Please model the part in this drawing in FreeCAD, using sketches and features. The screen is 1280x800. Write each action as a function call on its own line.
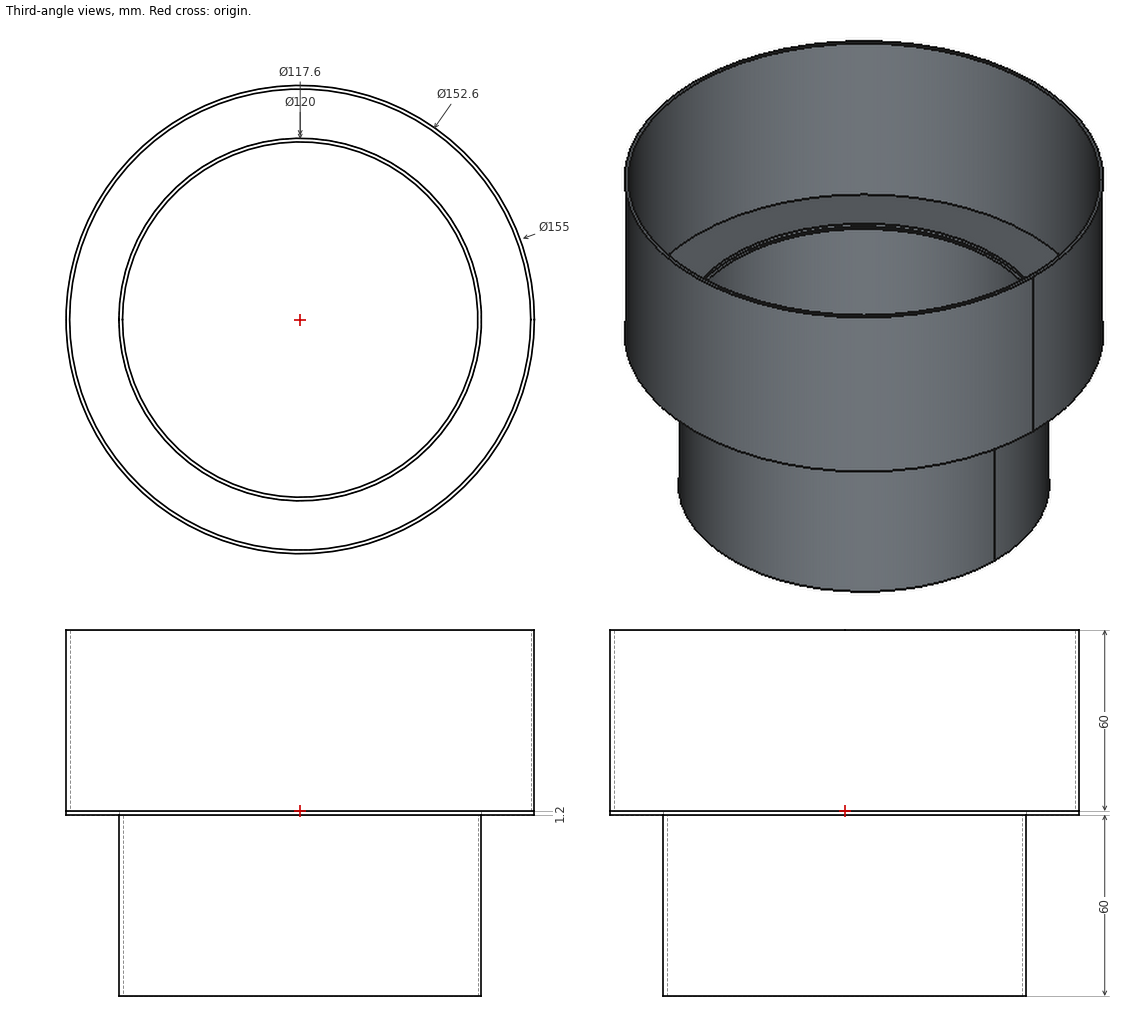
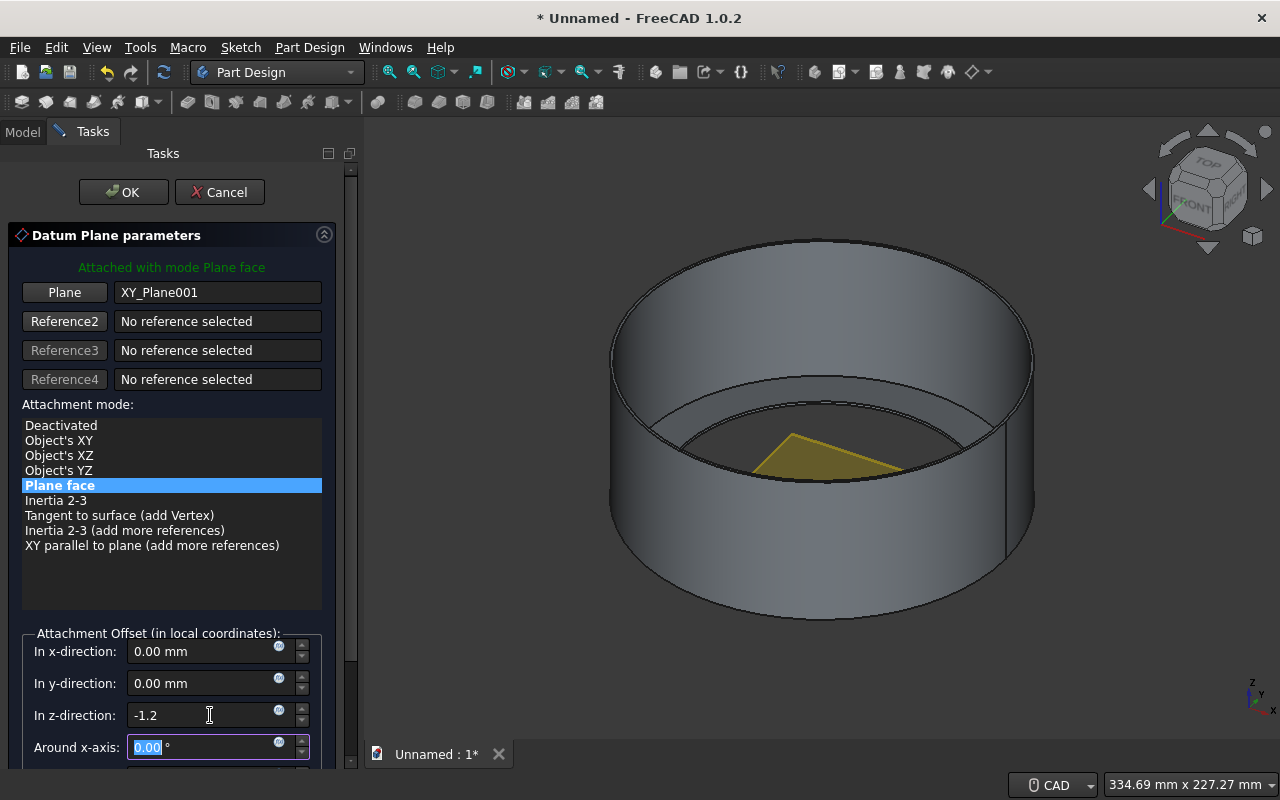
click(124, 192)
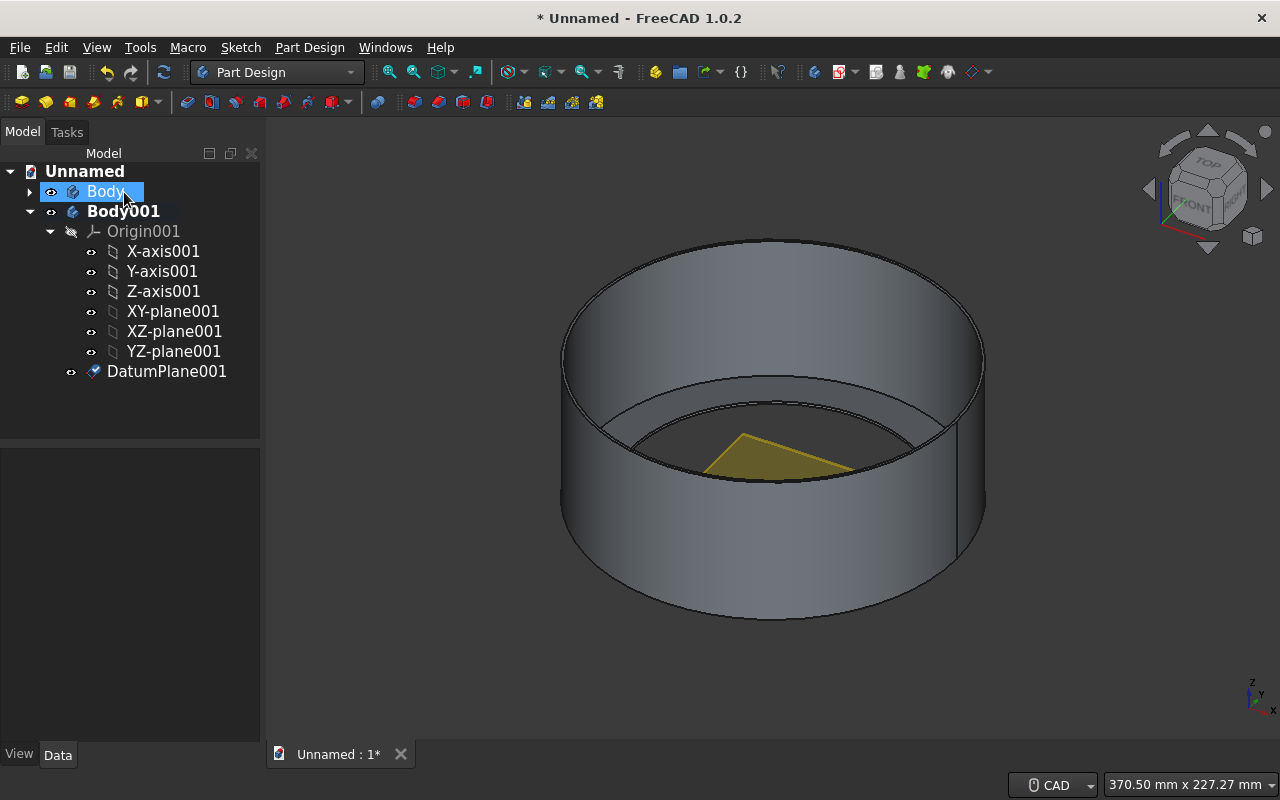
click(116, 372)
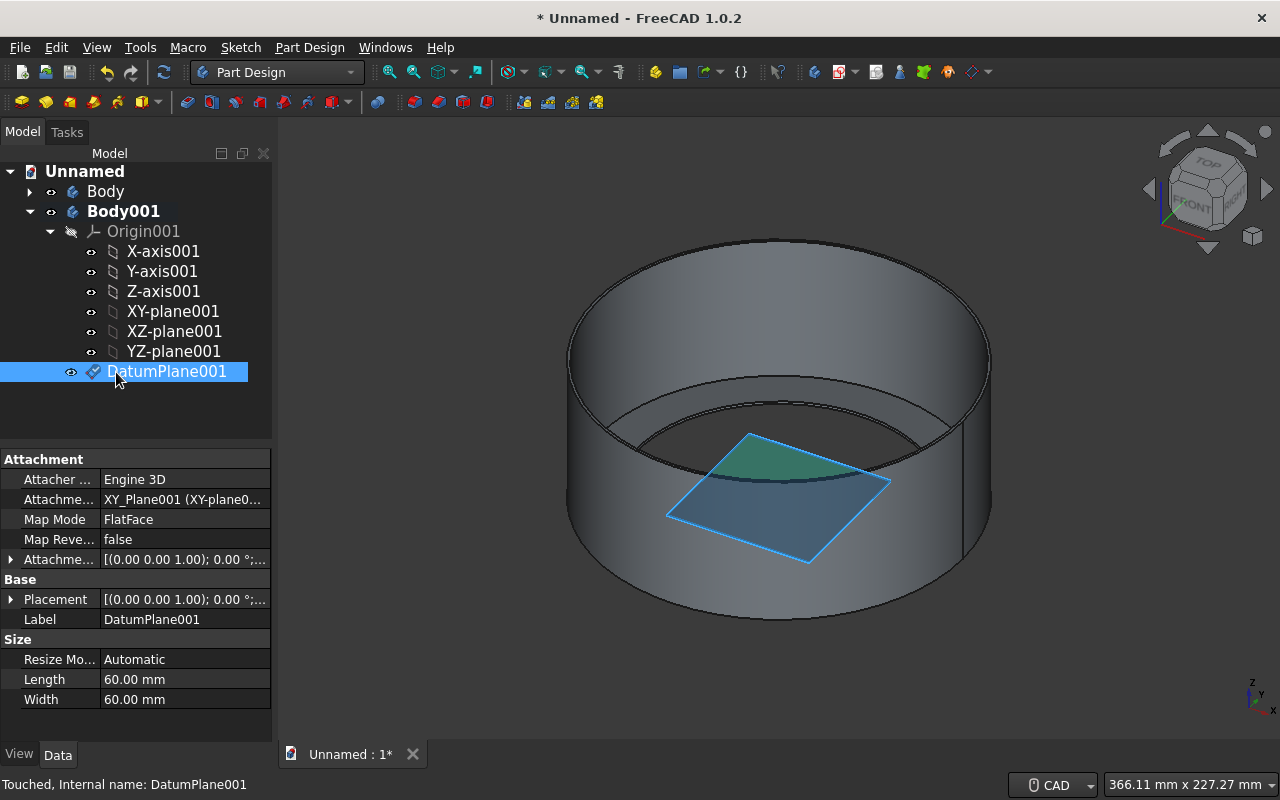
click(840, 72)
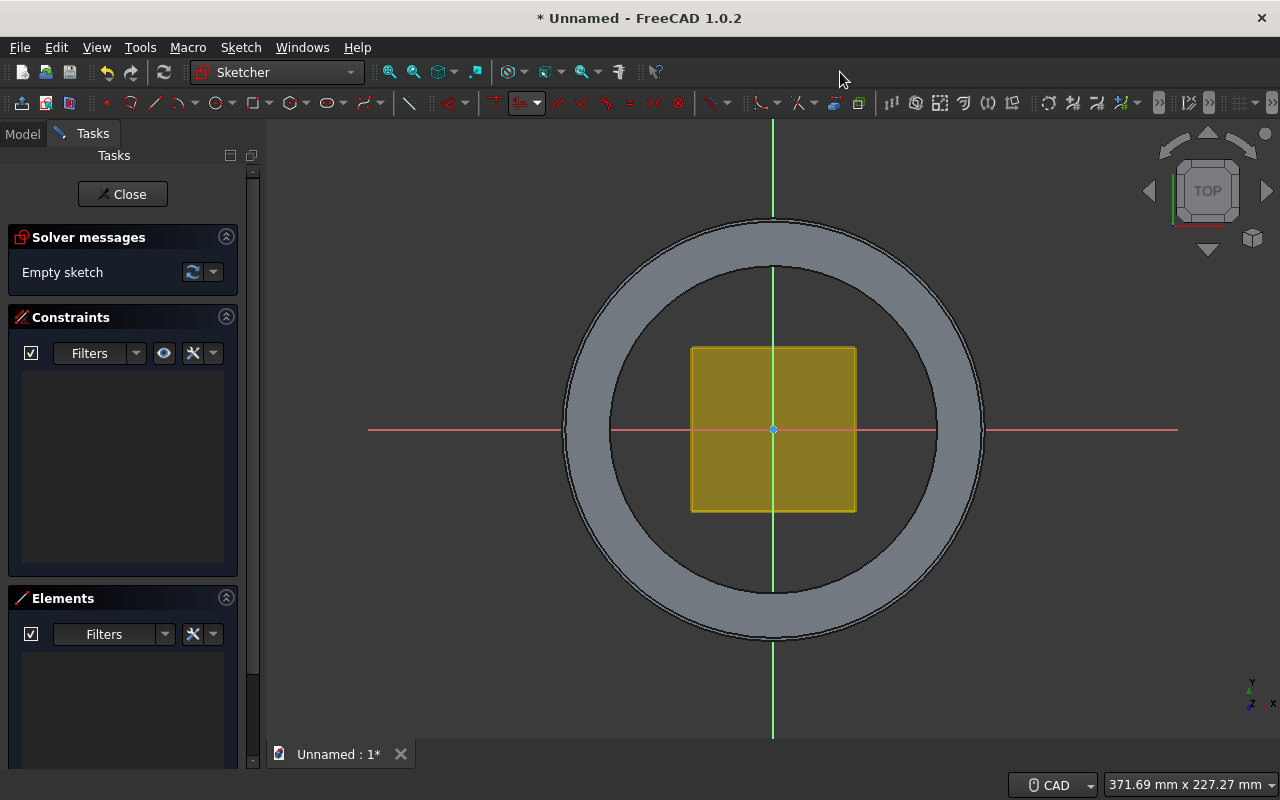
click(216, 104)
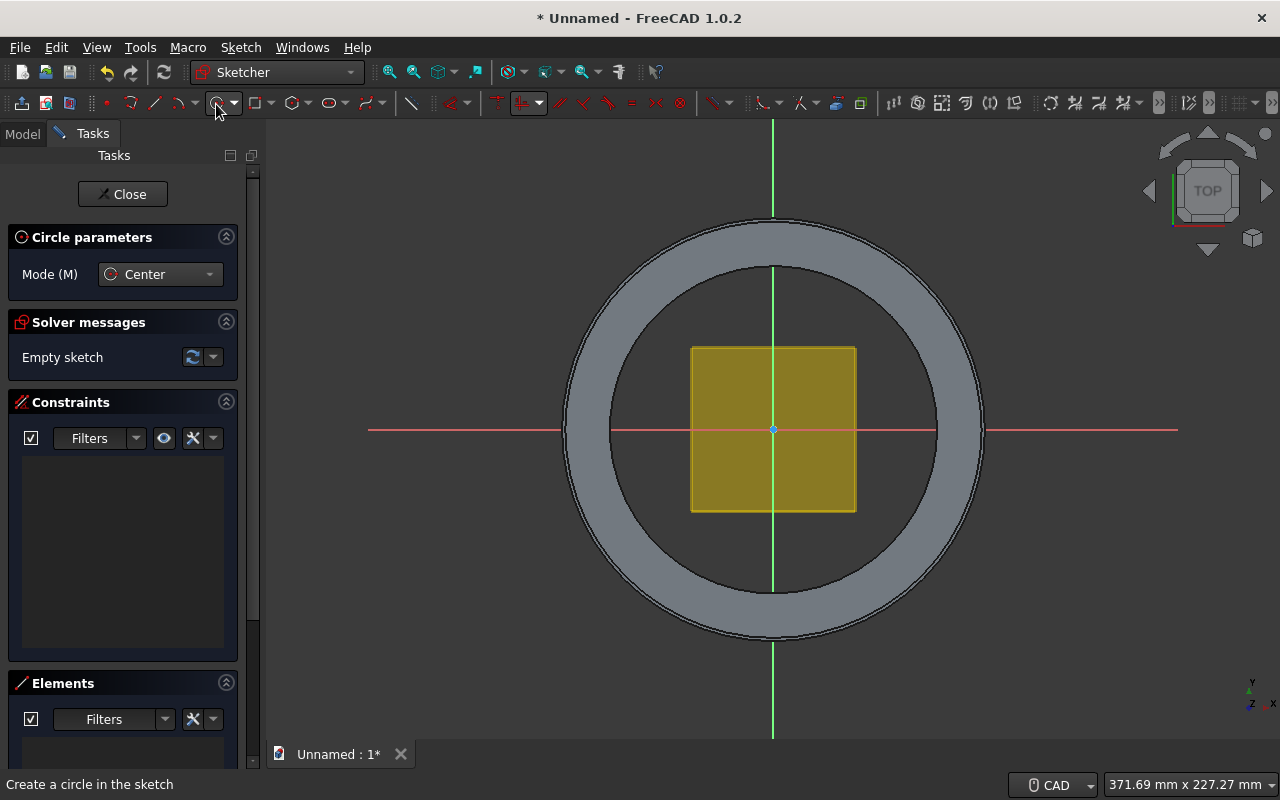
click(773, 430)
click(889, 314)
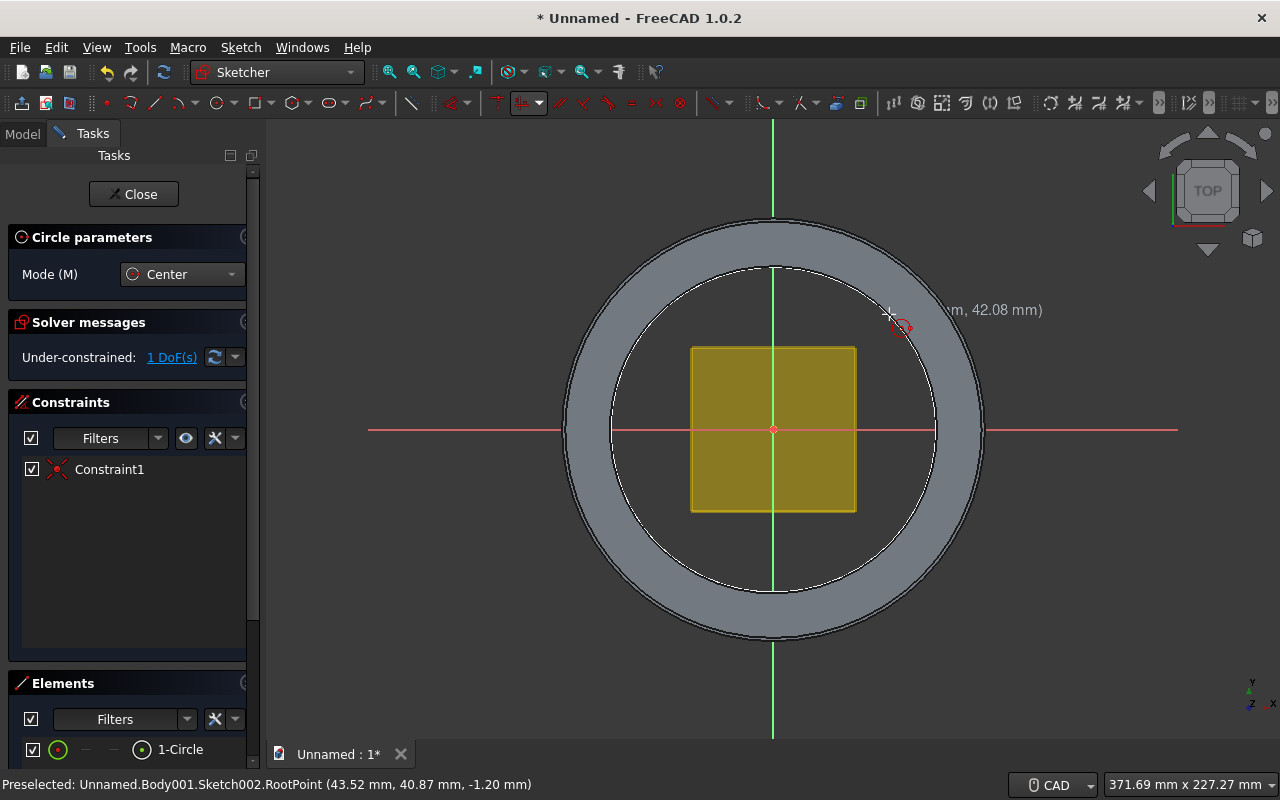
click(773, 430)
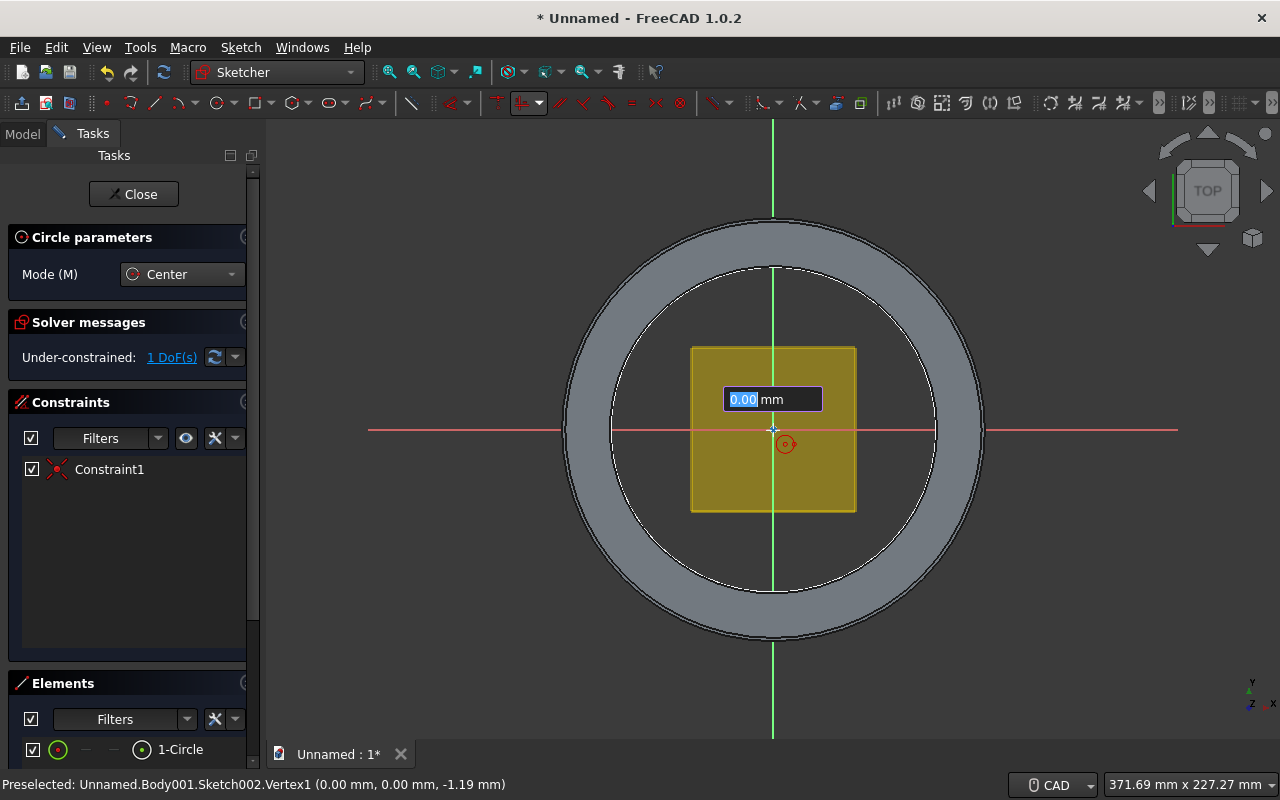
scroll(887, 316, up, 8)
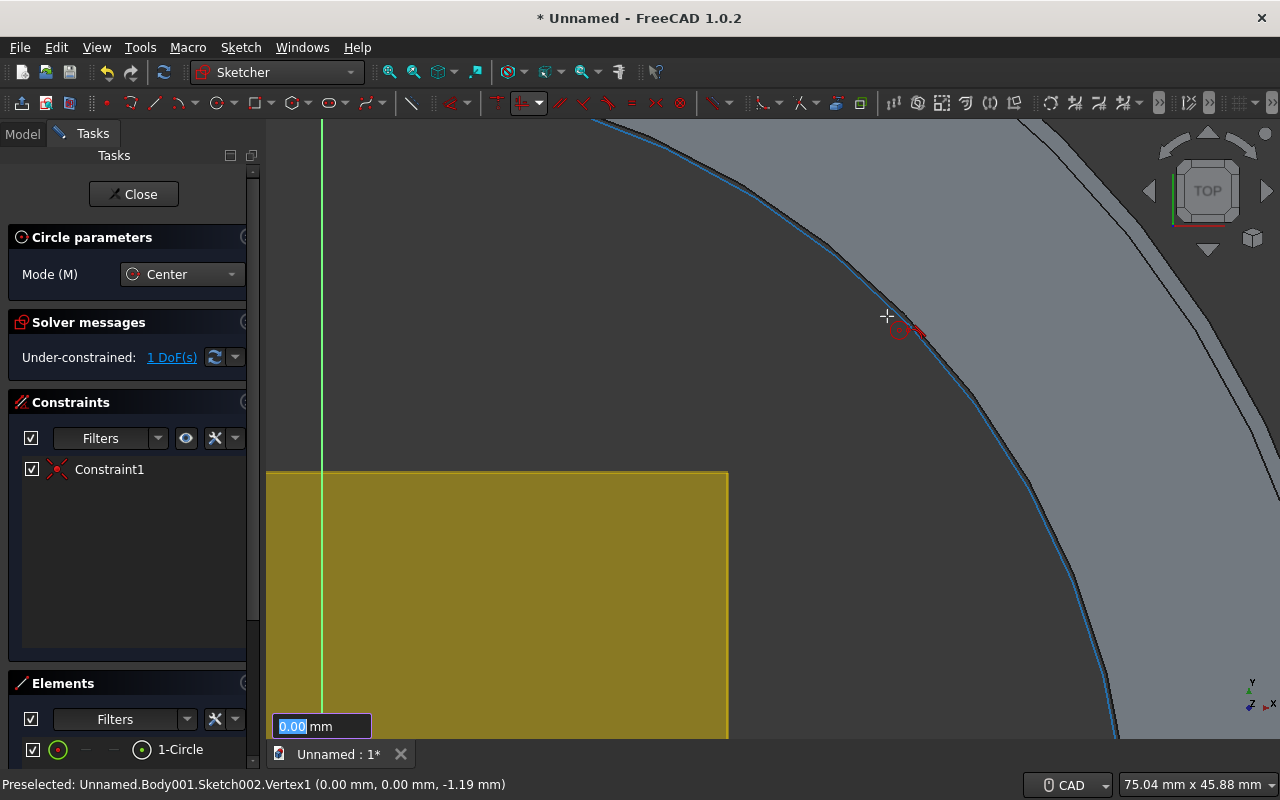
click(884, 317)
key(Escape)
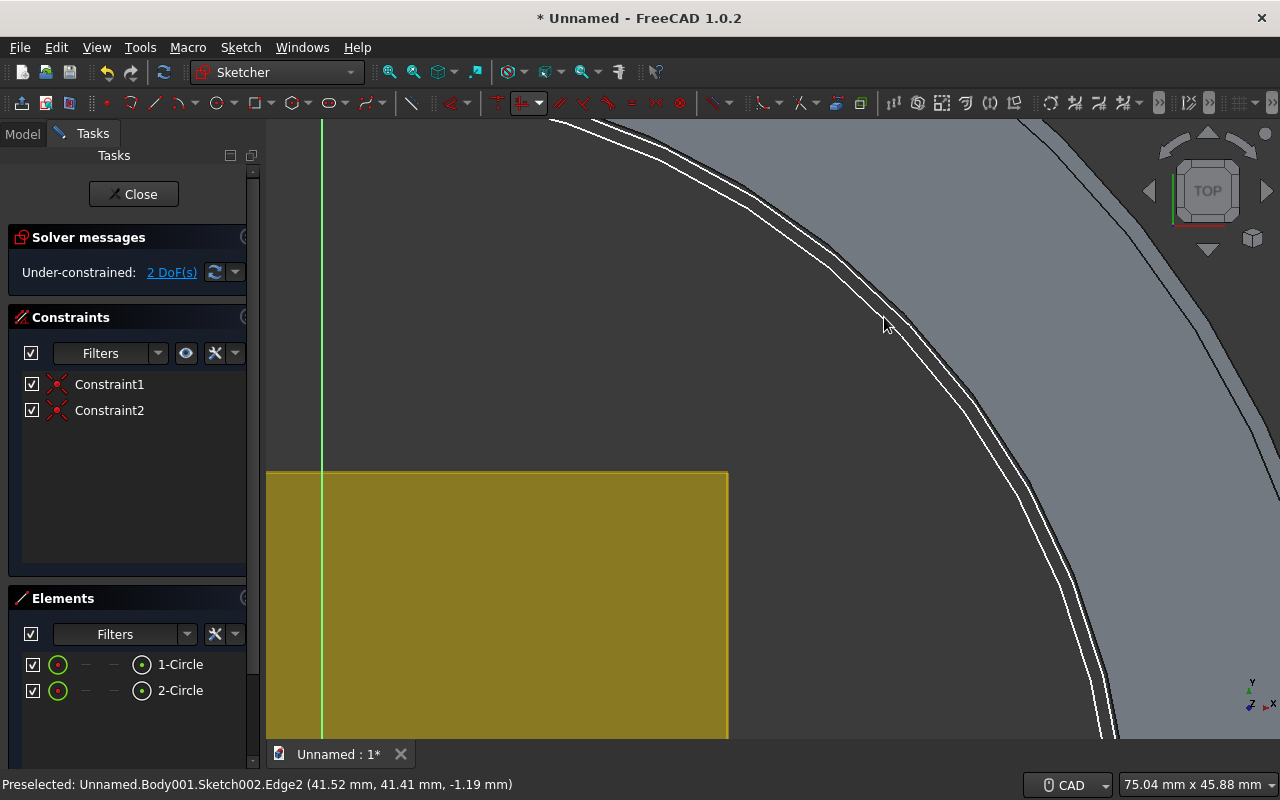
click(450, 104)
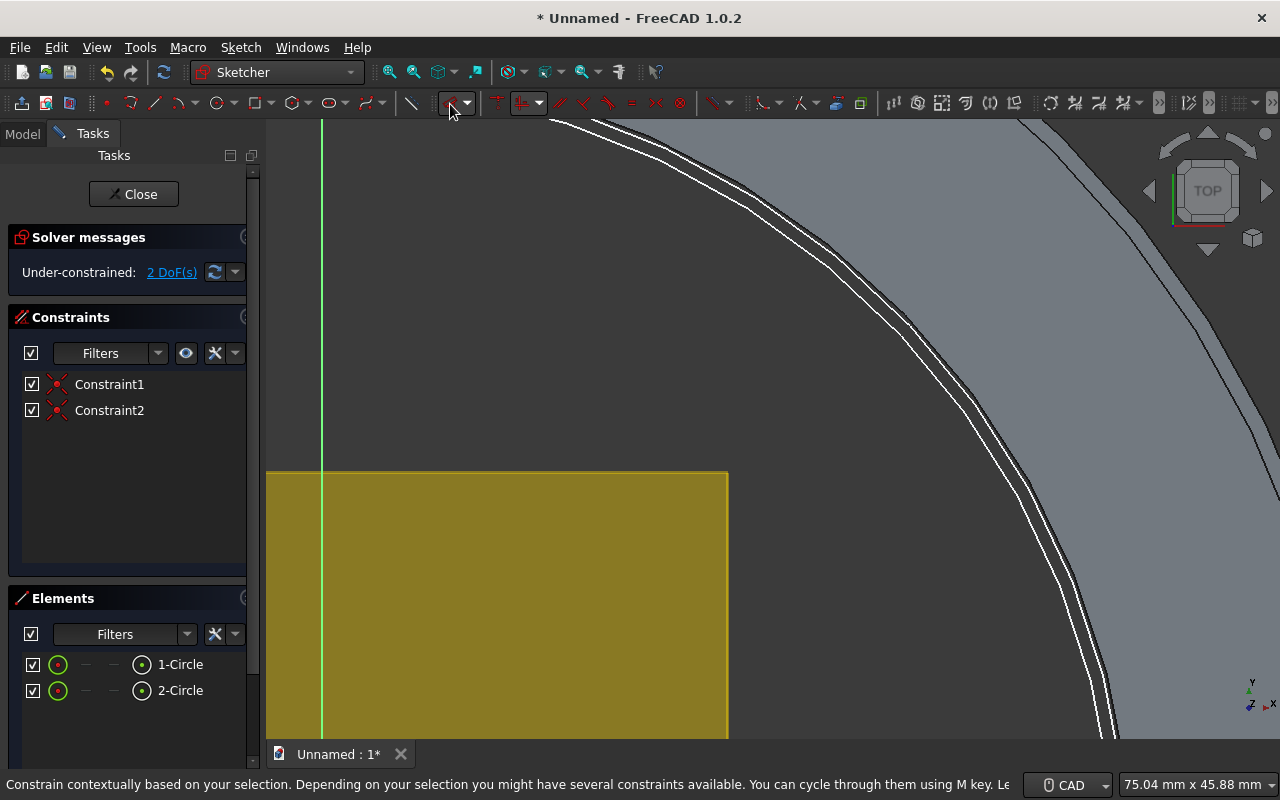
click(891, 306)
click(914, 283)